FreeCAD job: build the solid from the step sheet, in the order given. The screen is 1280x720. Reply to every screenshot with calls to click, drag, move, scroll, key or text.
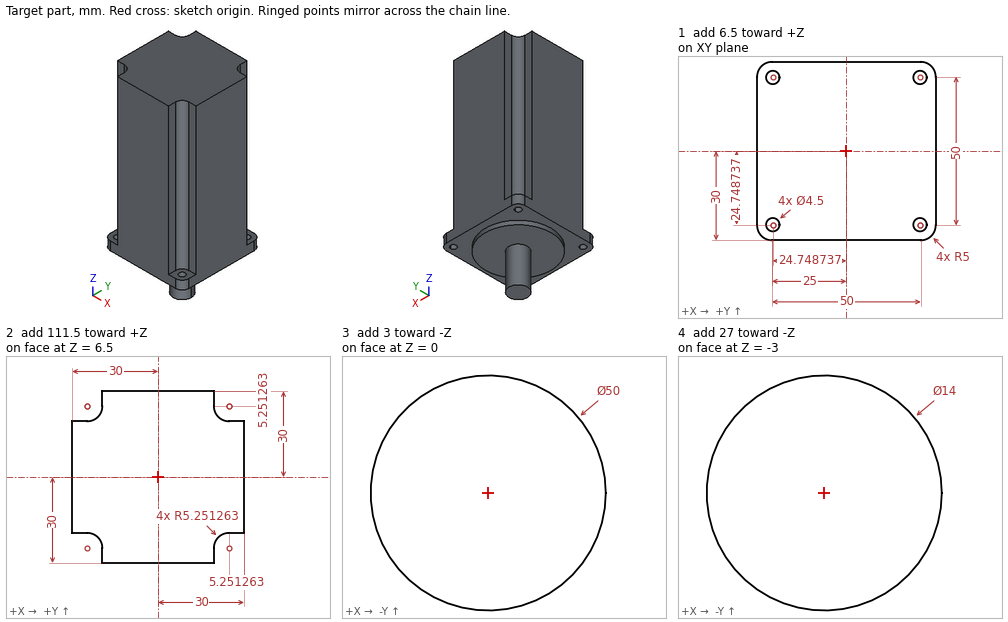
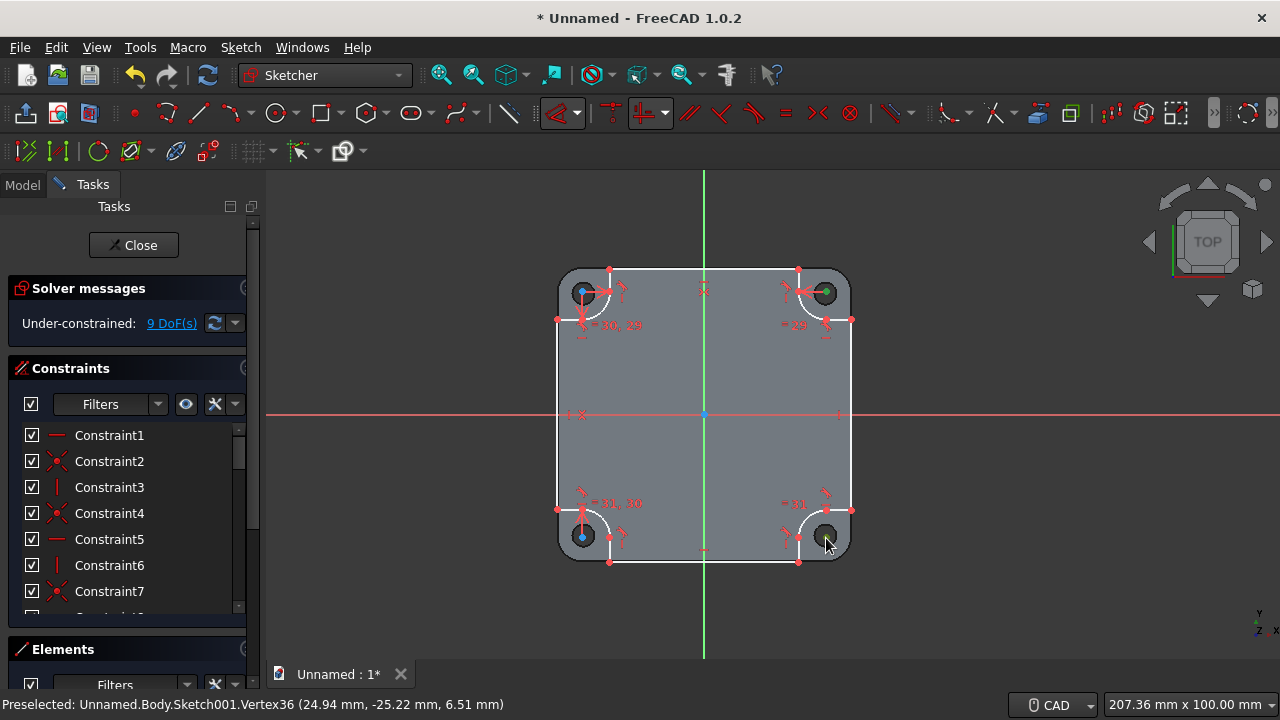
click(353, 415)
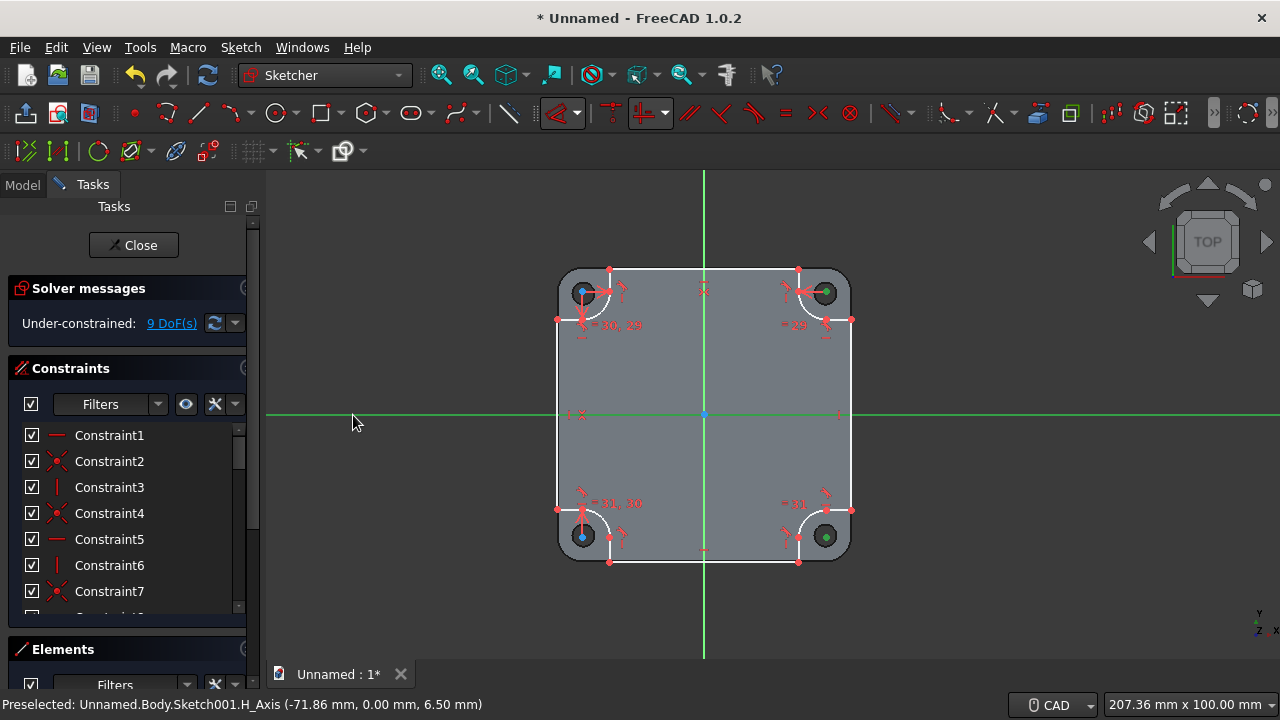
key(s)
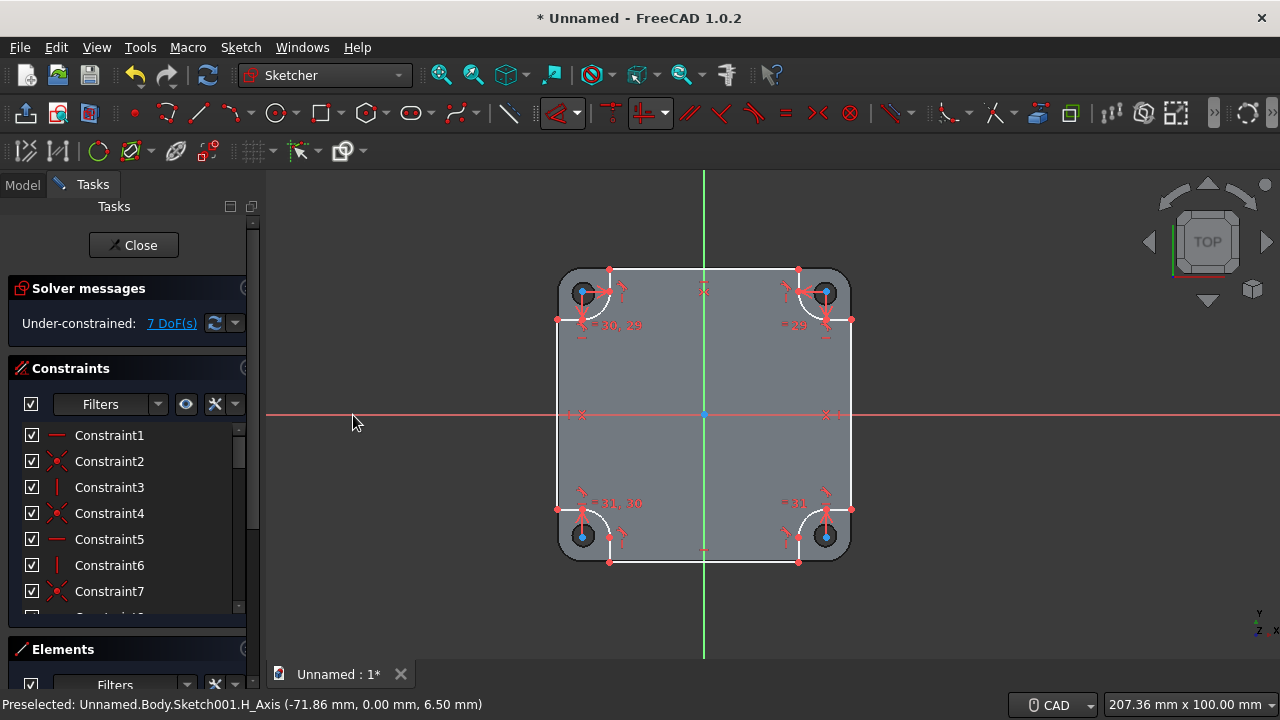
scroll(802, 304, up, 3)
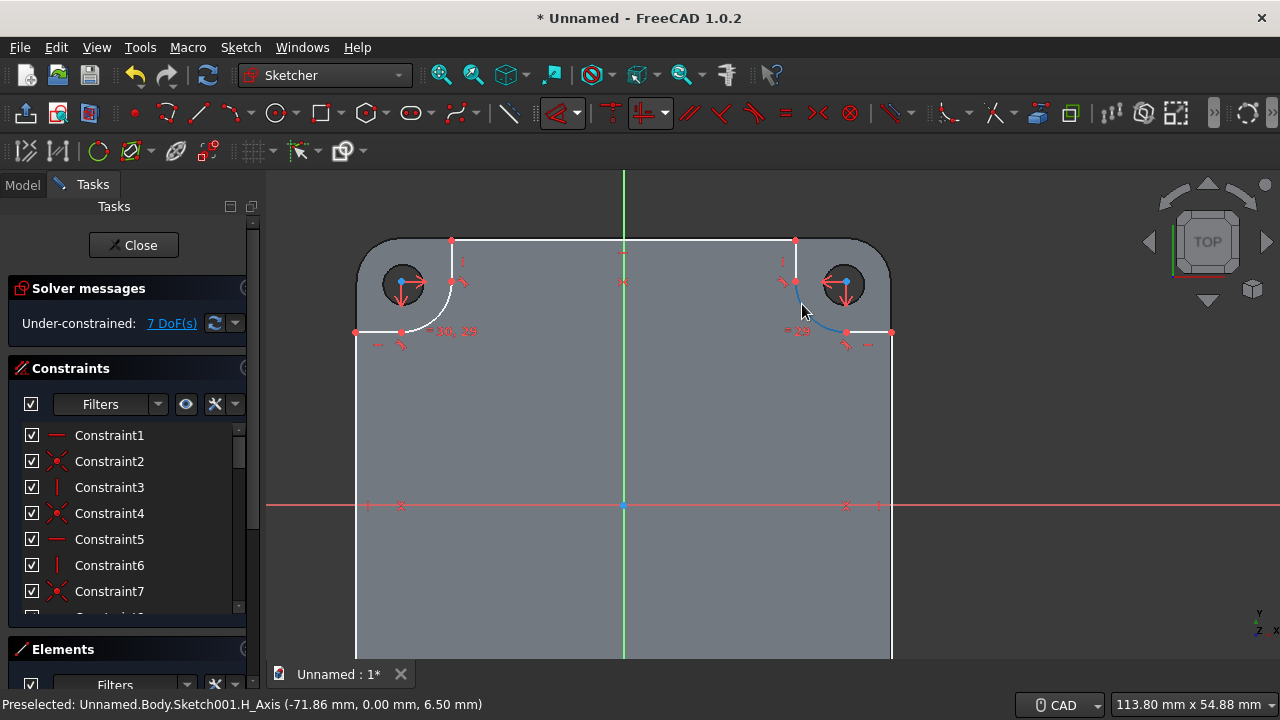
click(801, 305)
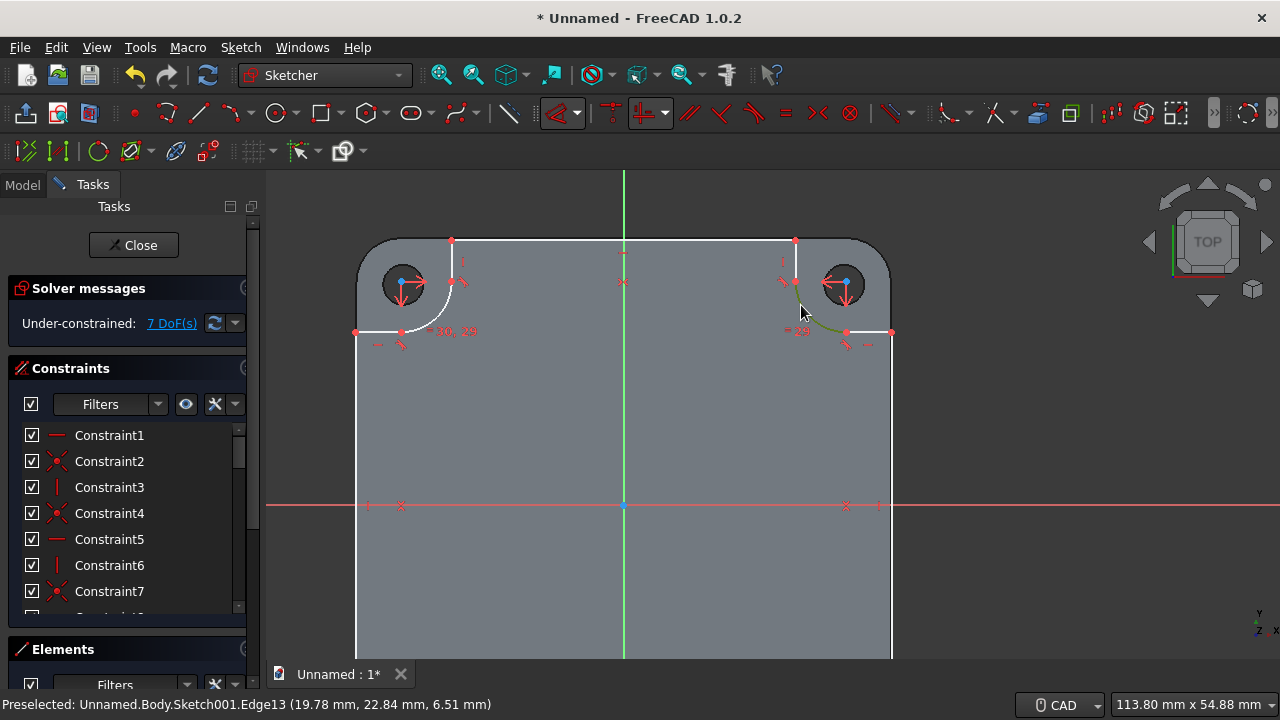
click(580, 114)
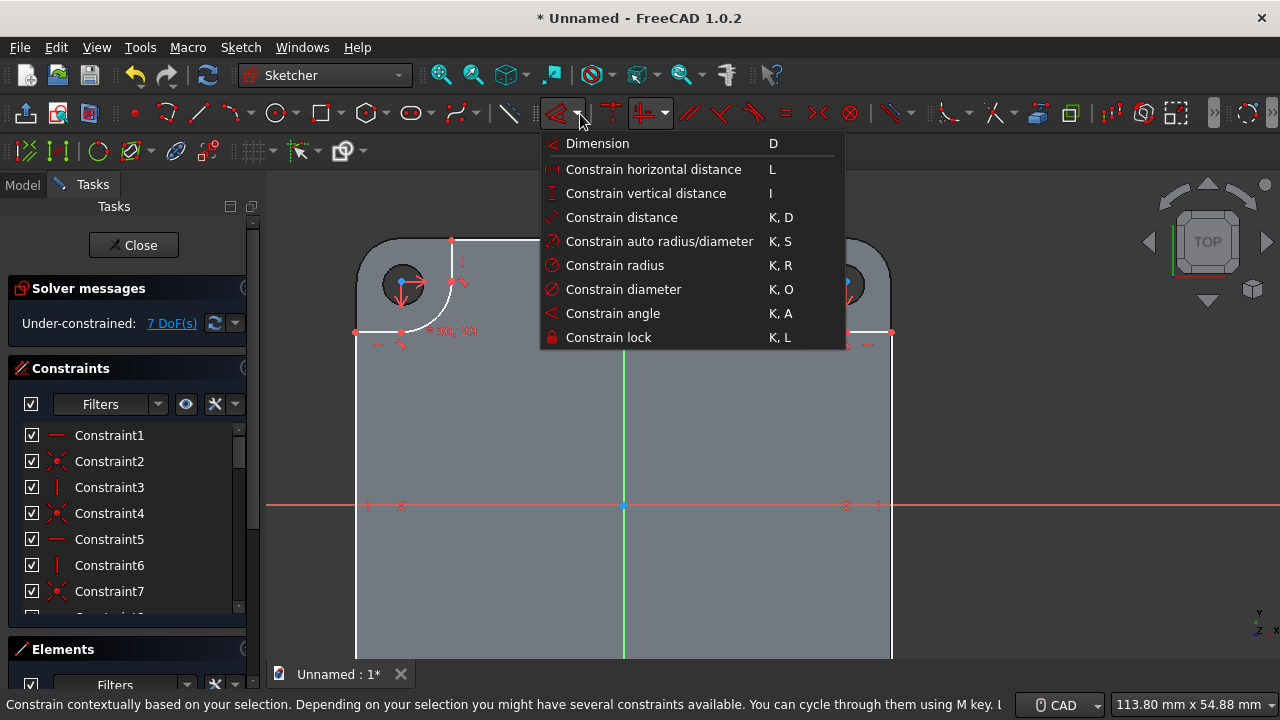
click(693, 265)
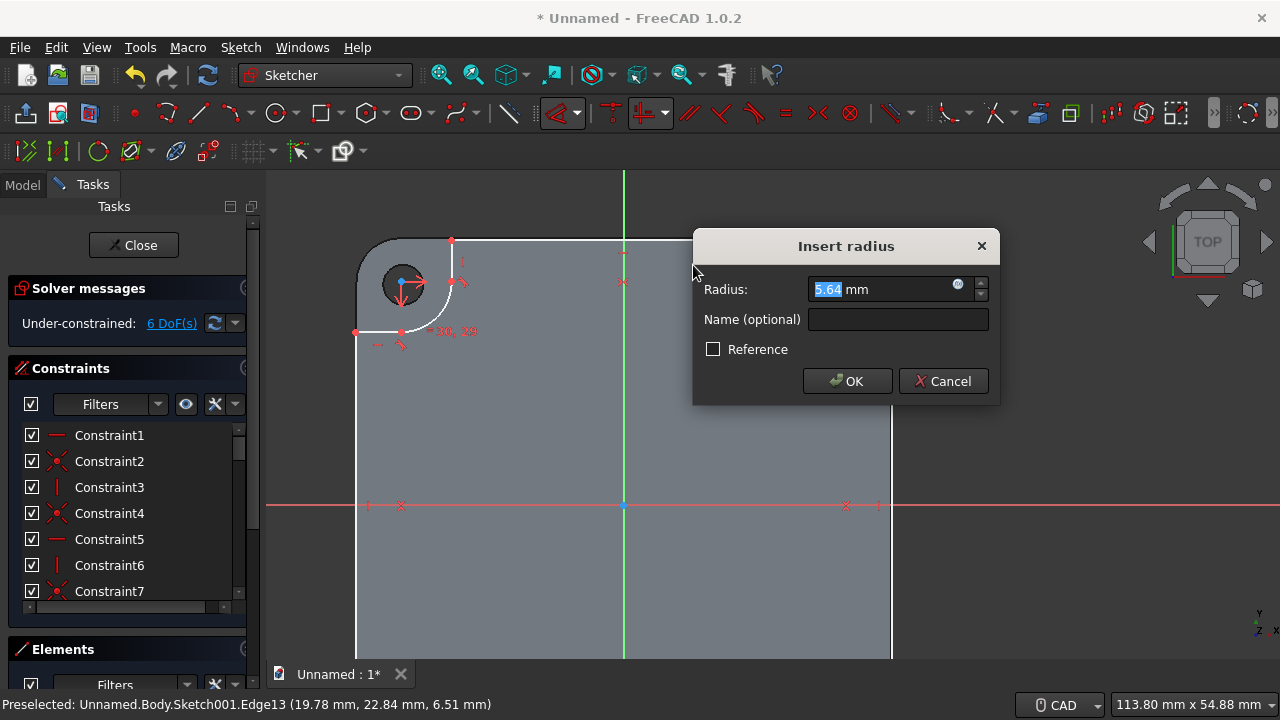
text(5.251263)
key(Return)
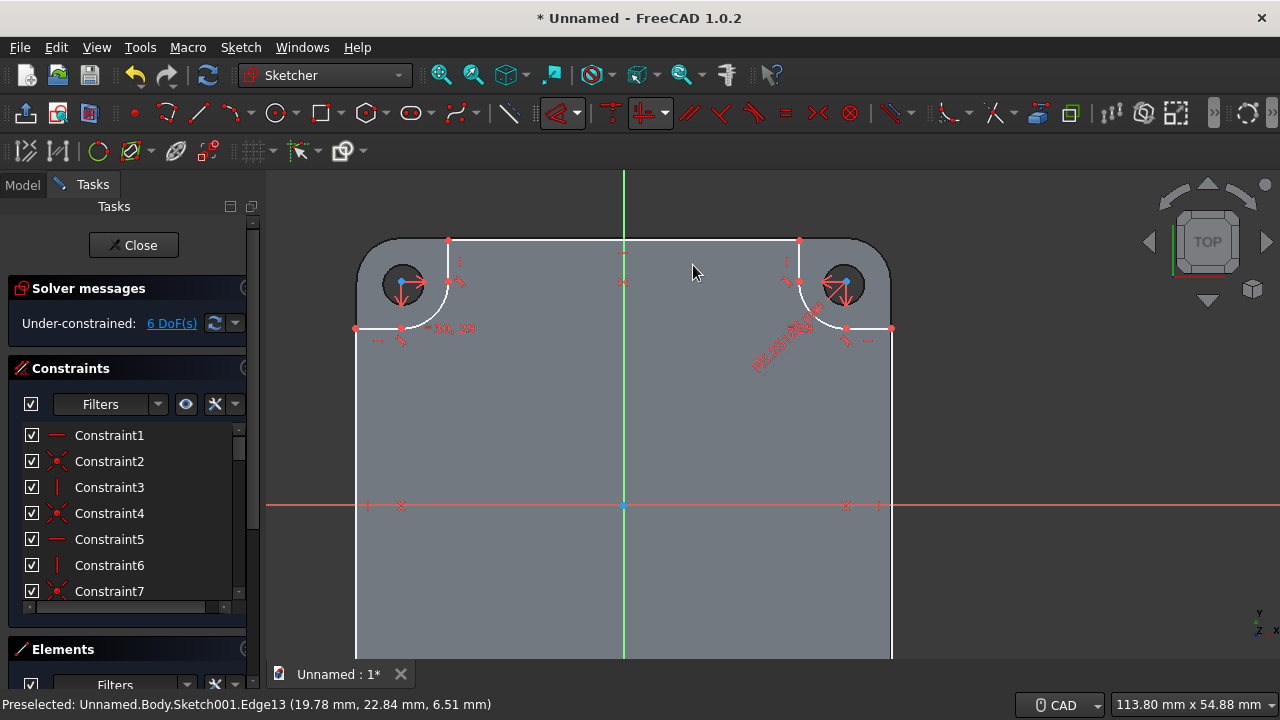
scroll(803, 304, down, 3)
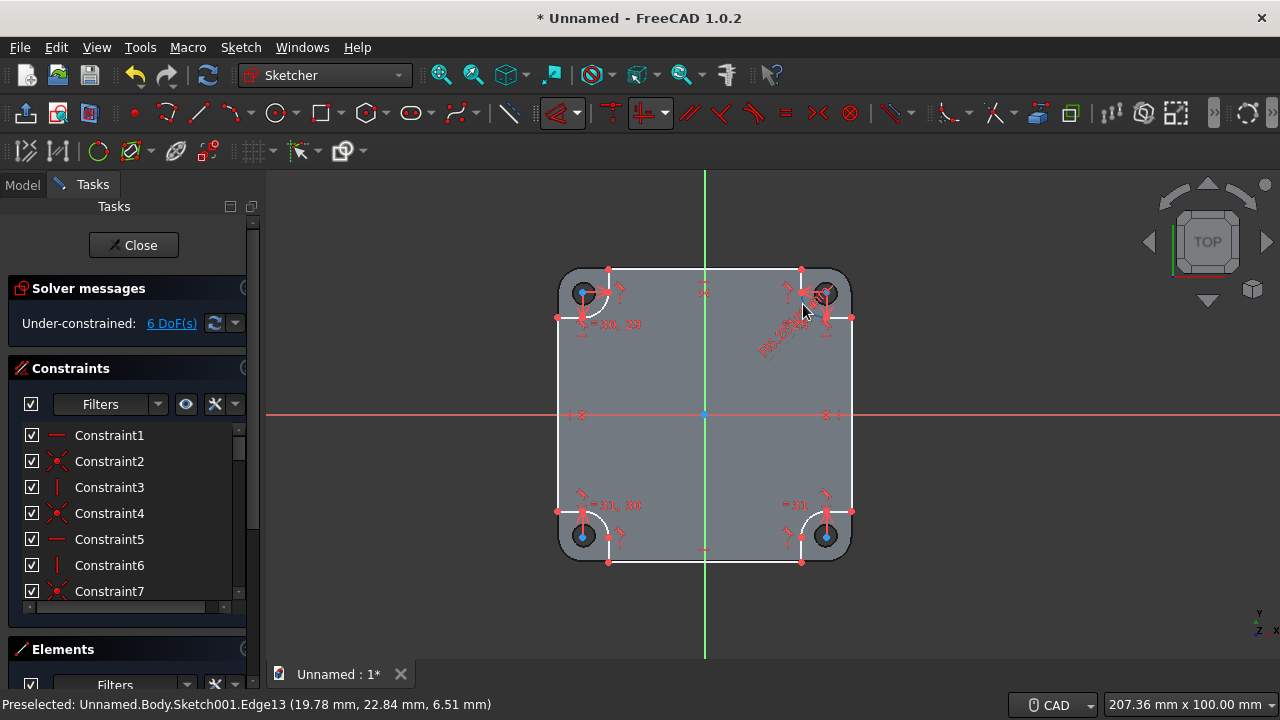
click(852, 512)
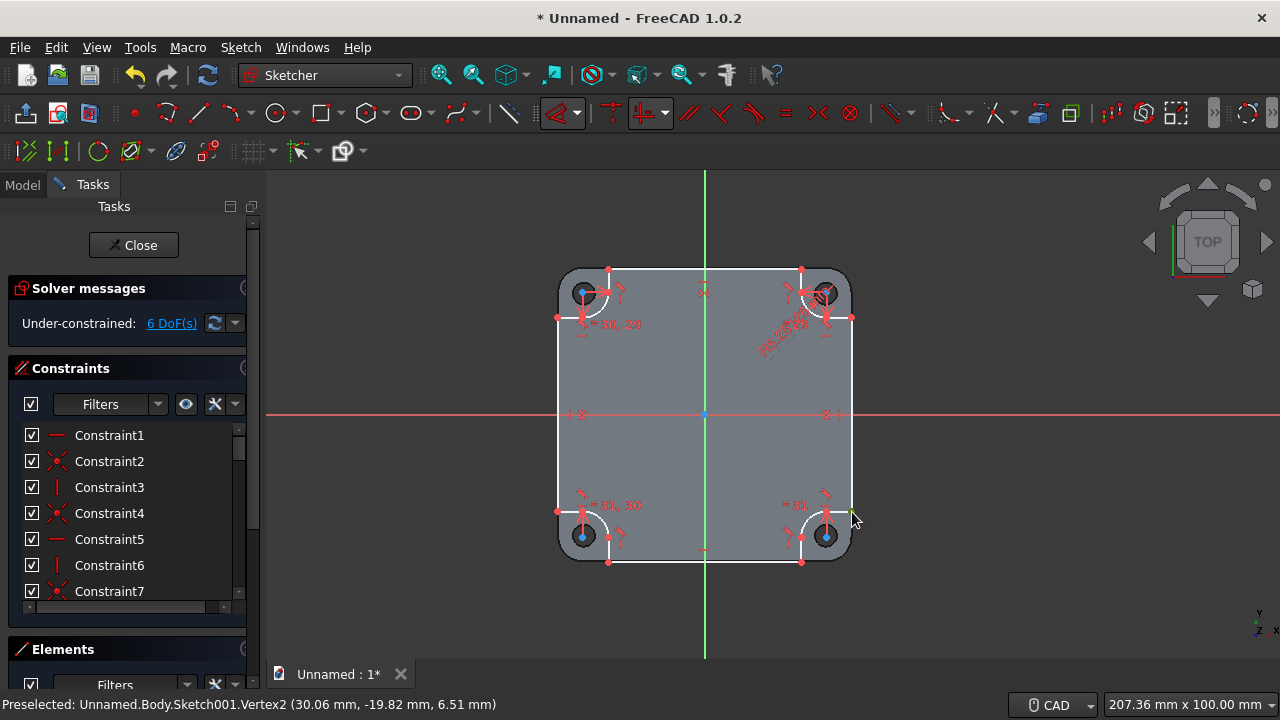
key(l)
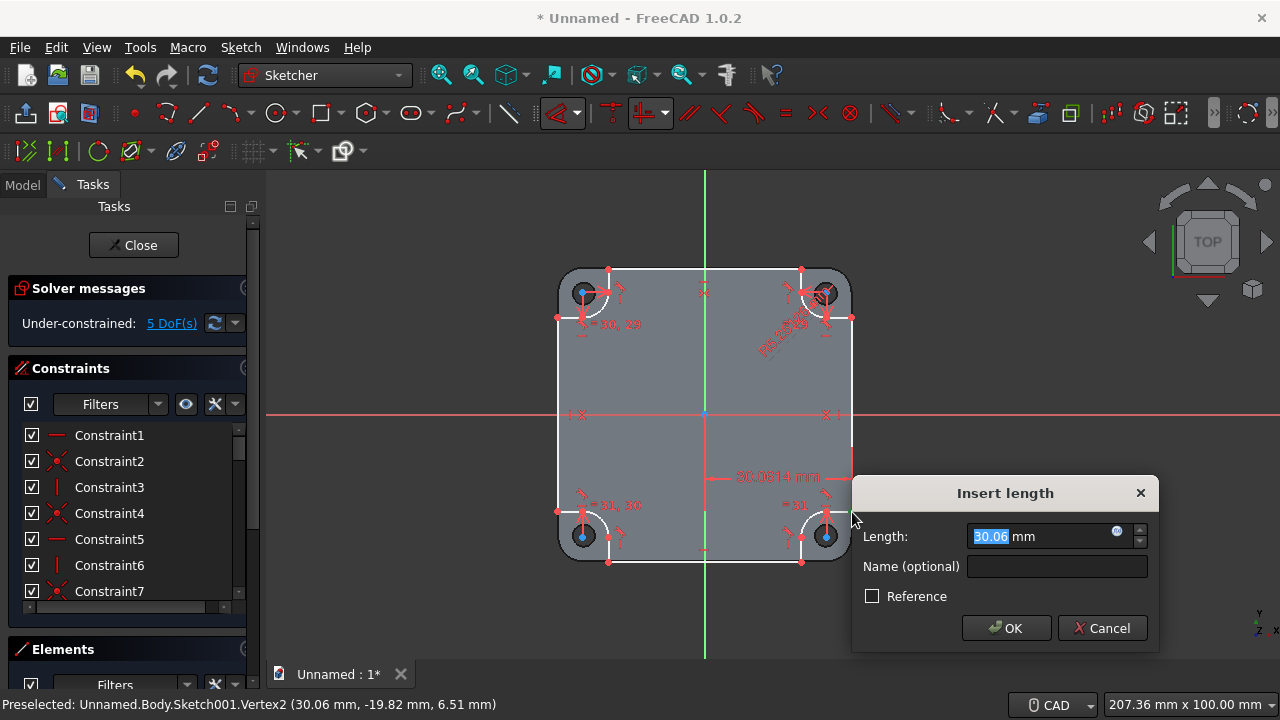
text(30)
key(Return)